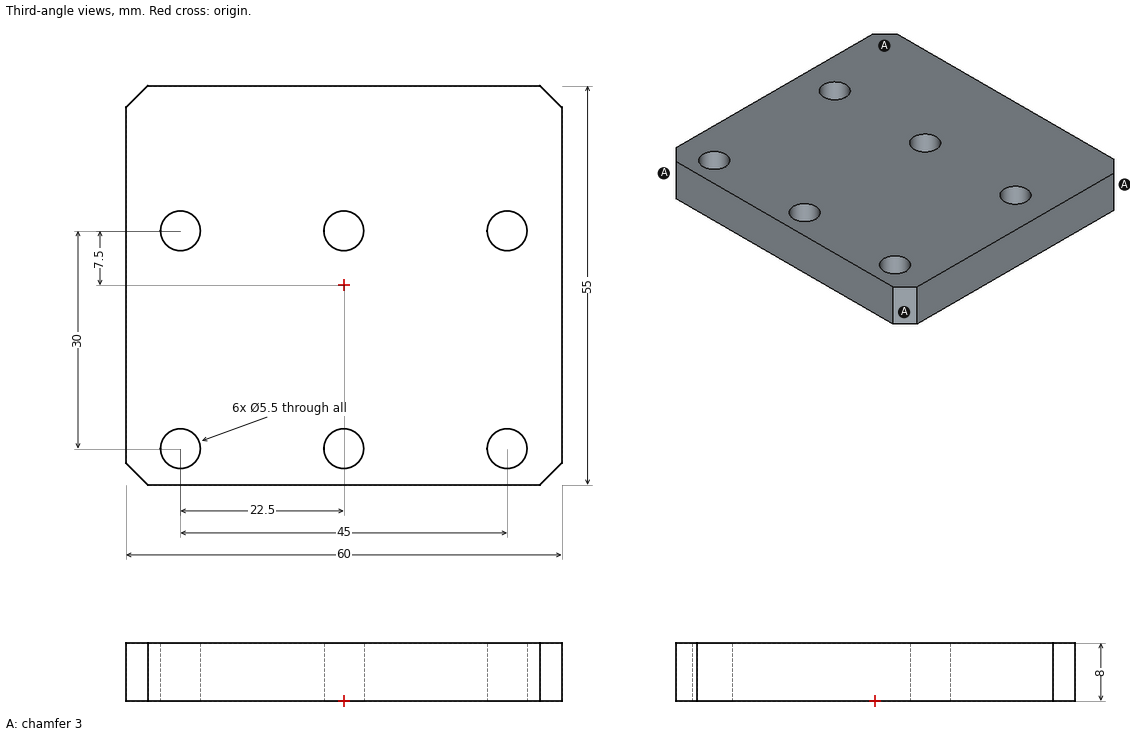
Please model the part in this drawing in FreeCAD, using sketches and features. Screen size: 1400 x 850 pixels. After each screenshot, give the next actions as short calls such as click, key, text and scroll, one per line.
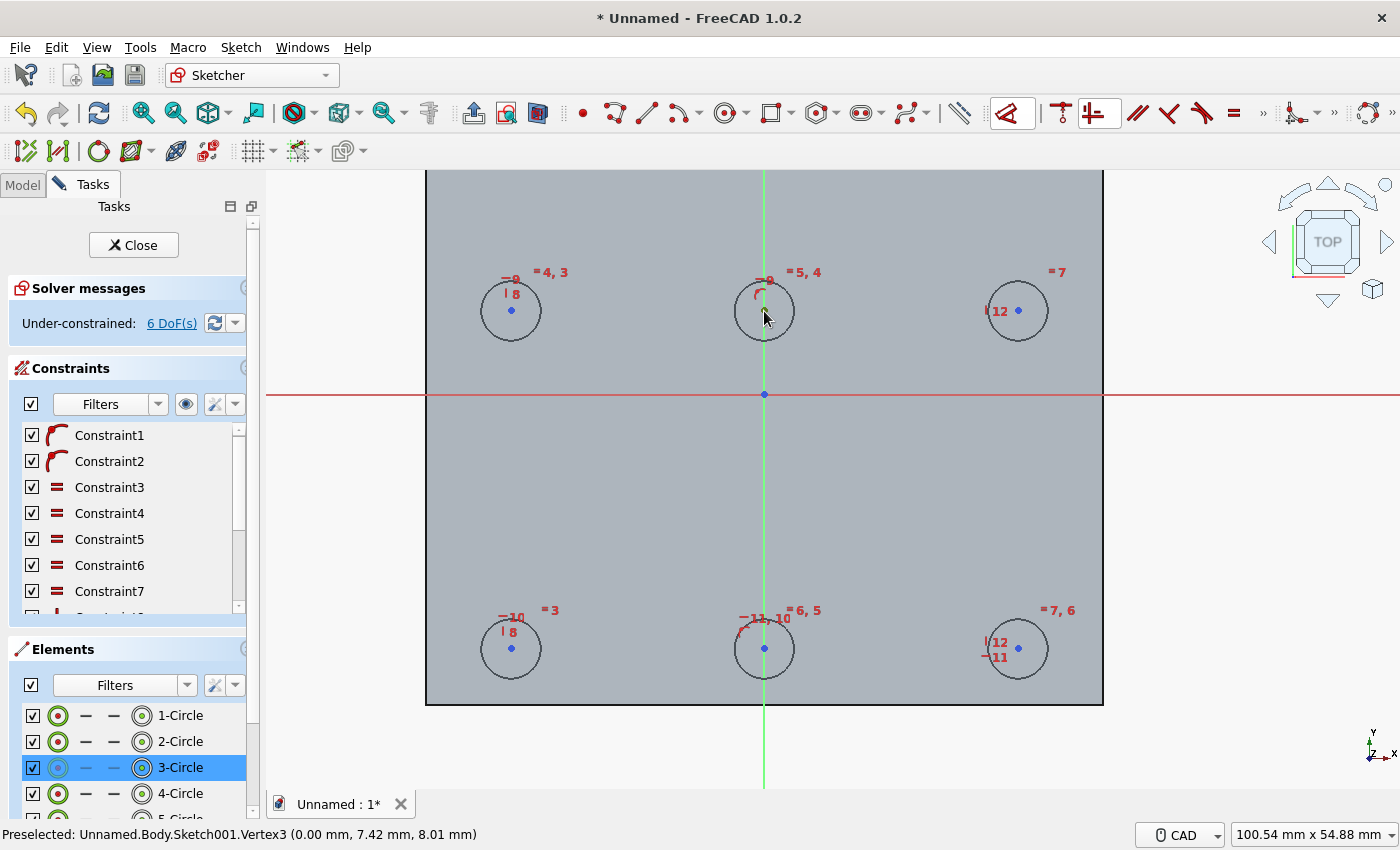
click(1018, 311)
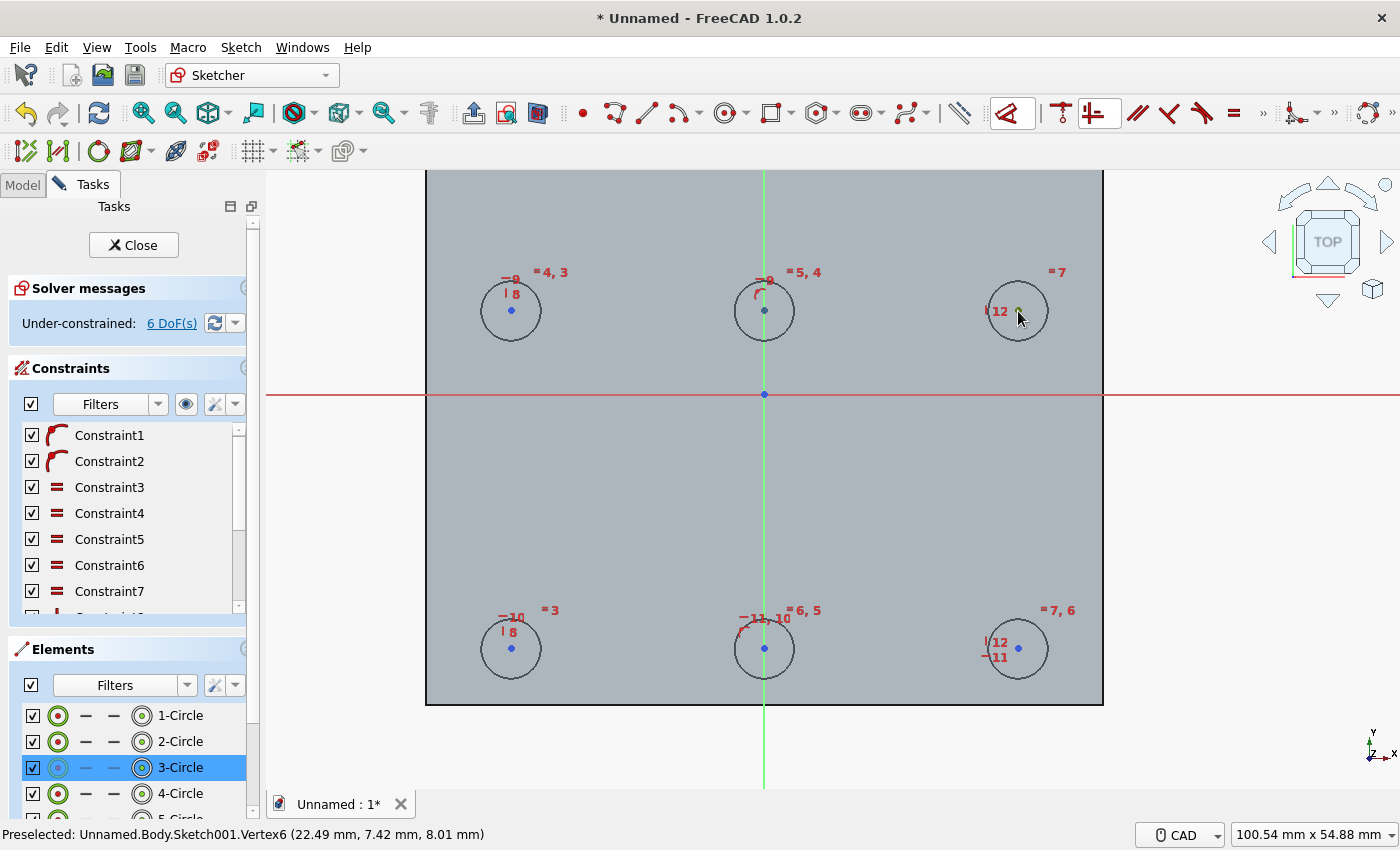
click(1116, 114)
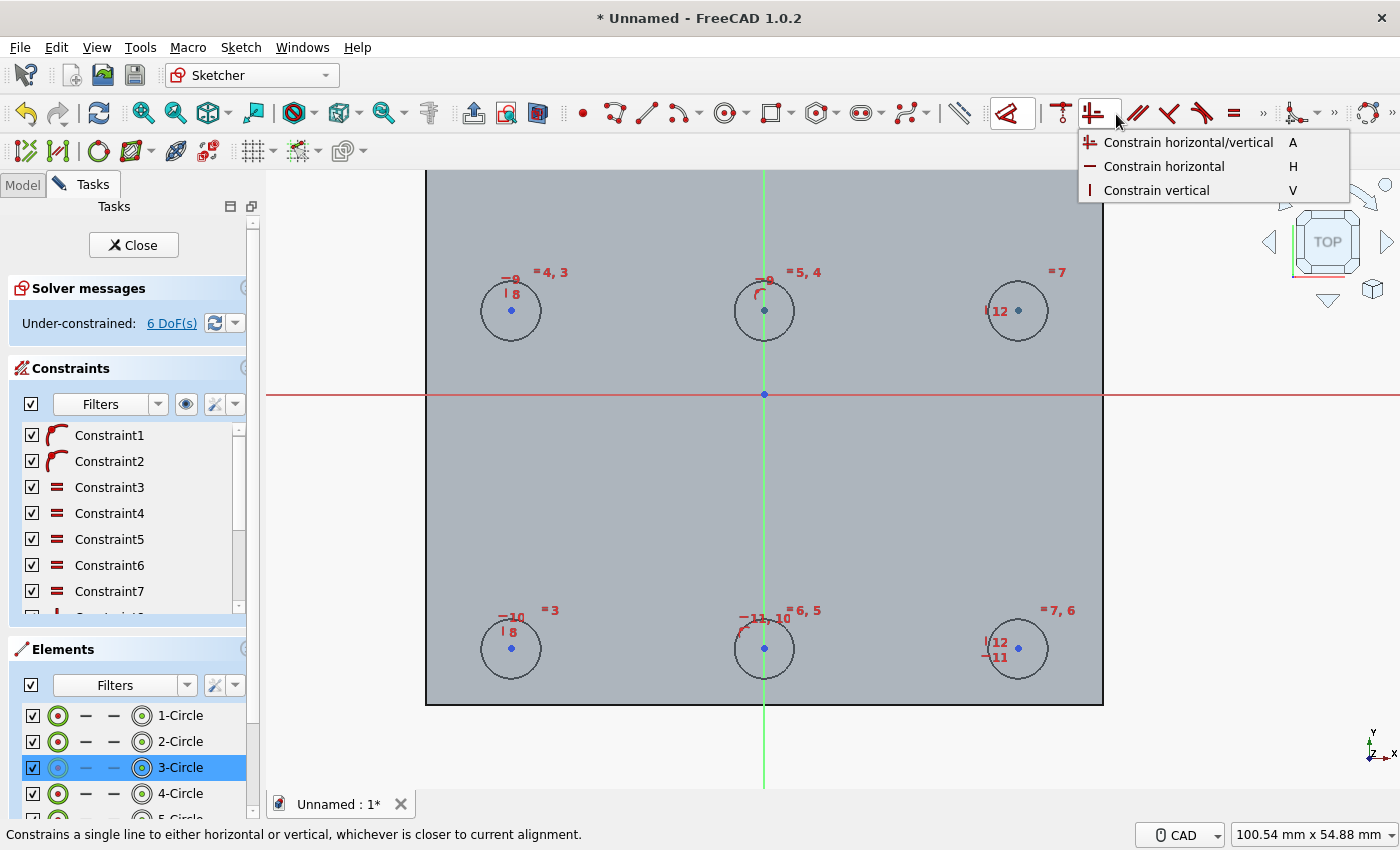
click(1214, 166)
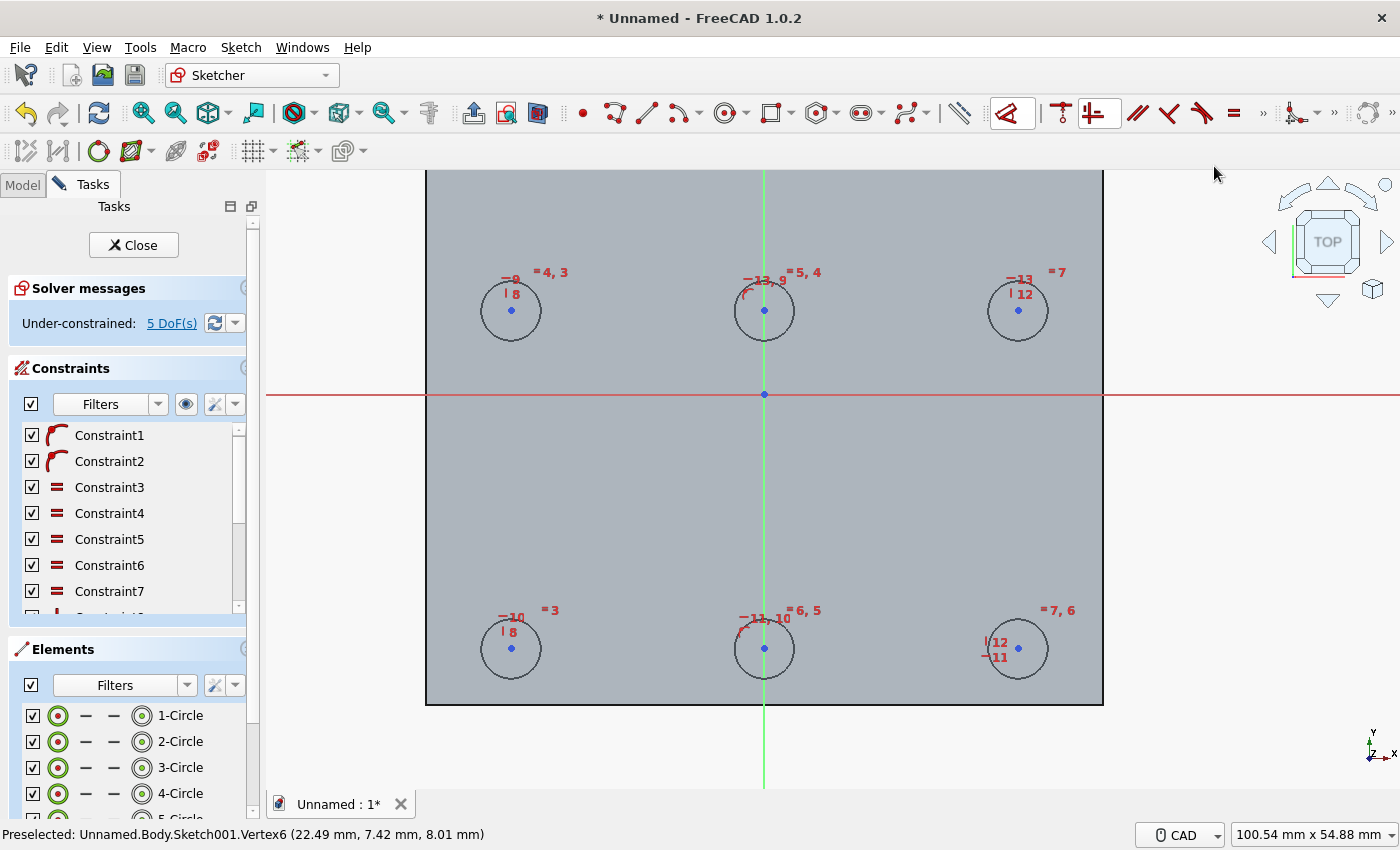
click(1006, 114)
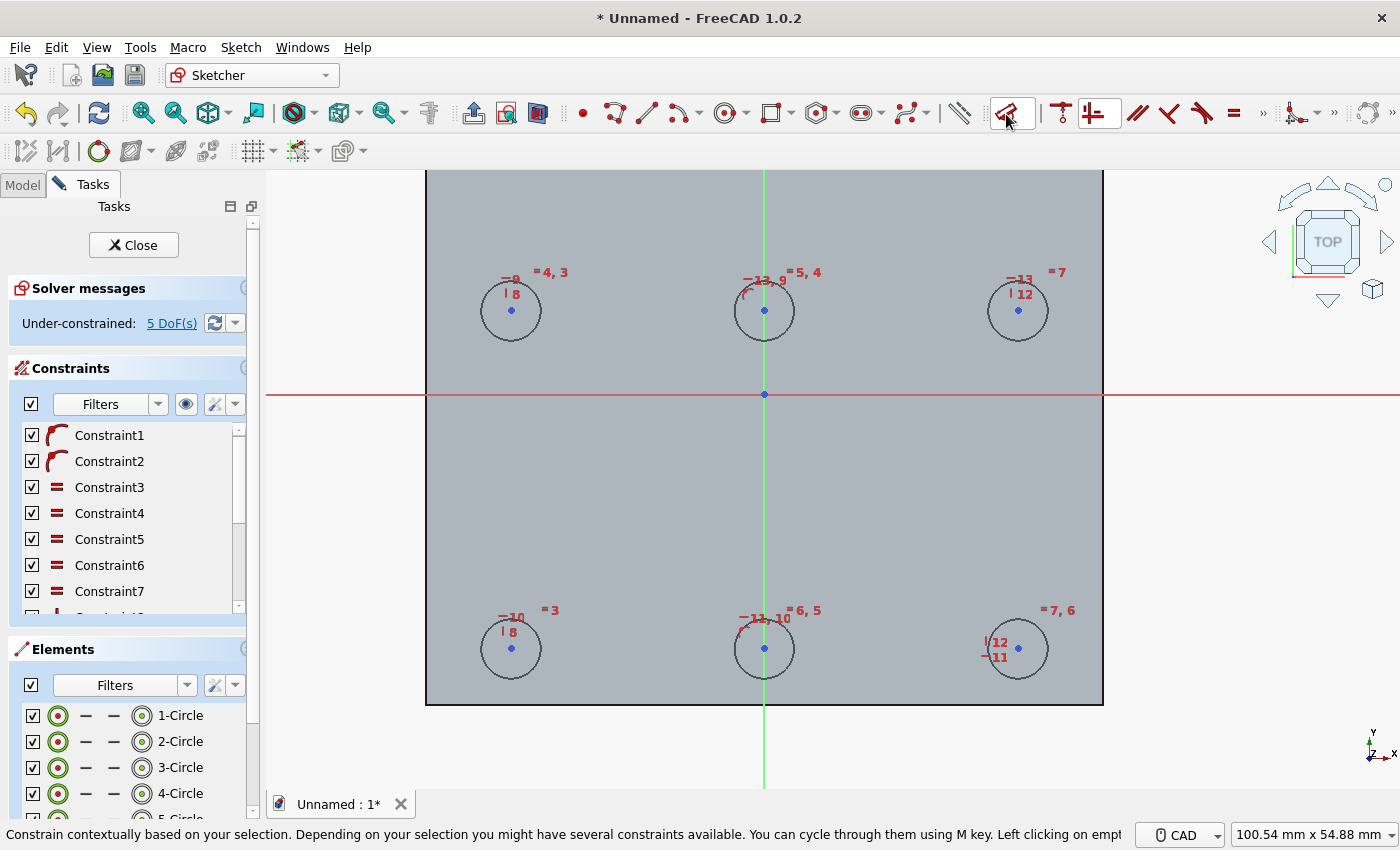
click(532, 628)
click(555, 605)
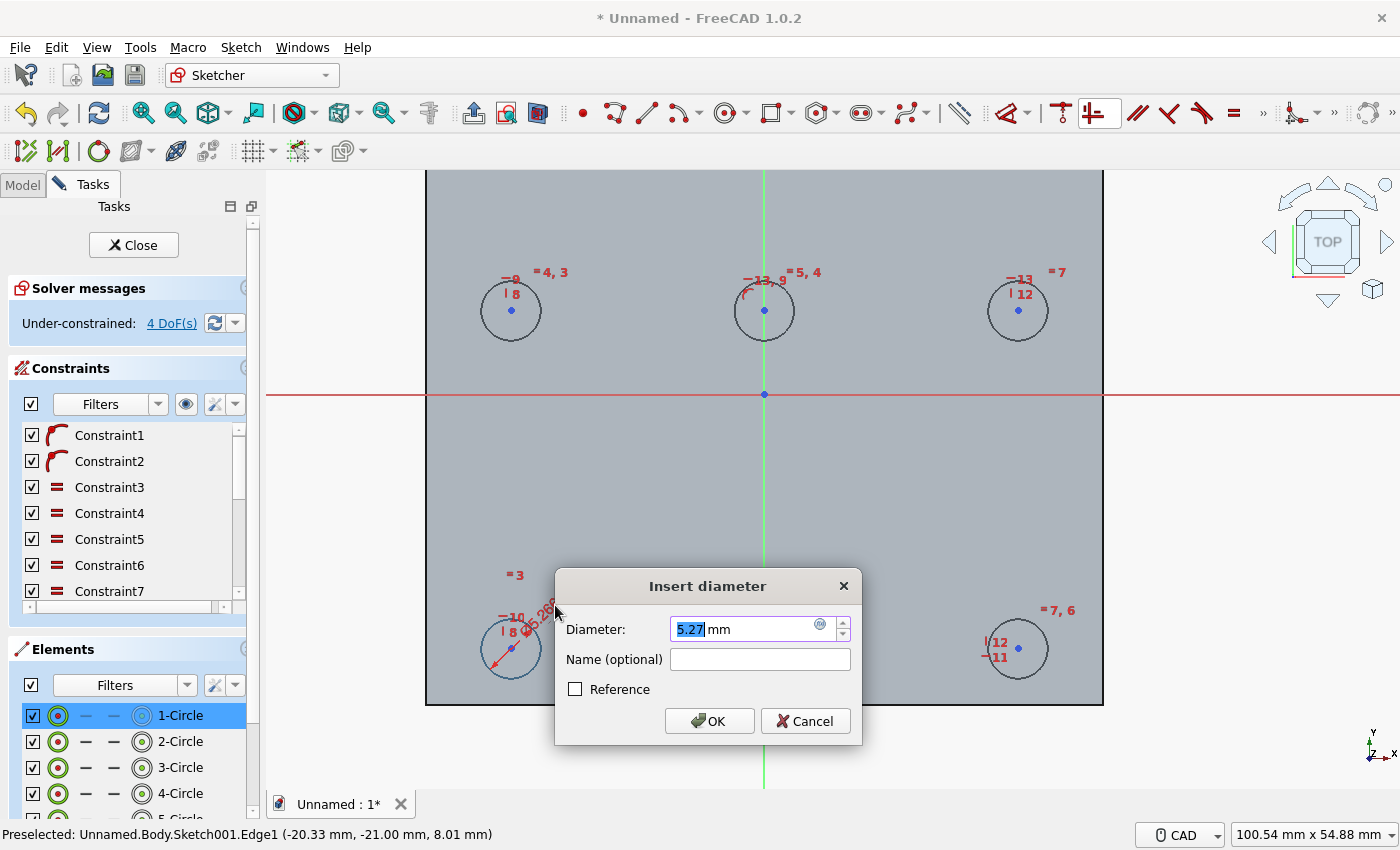
text(5.5)
key(Return)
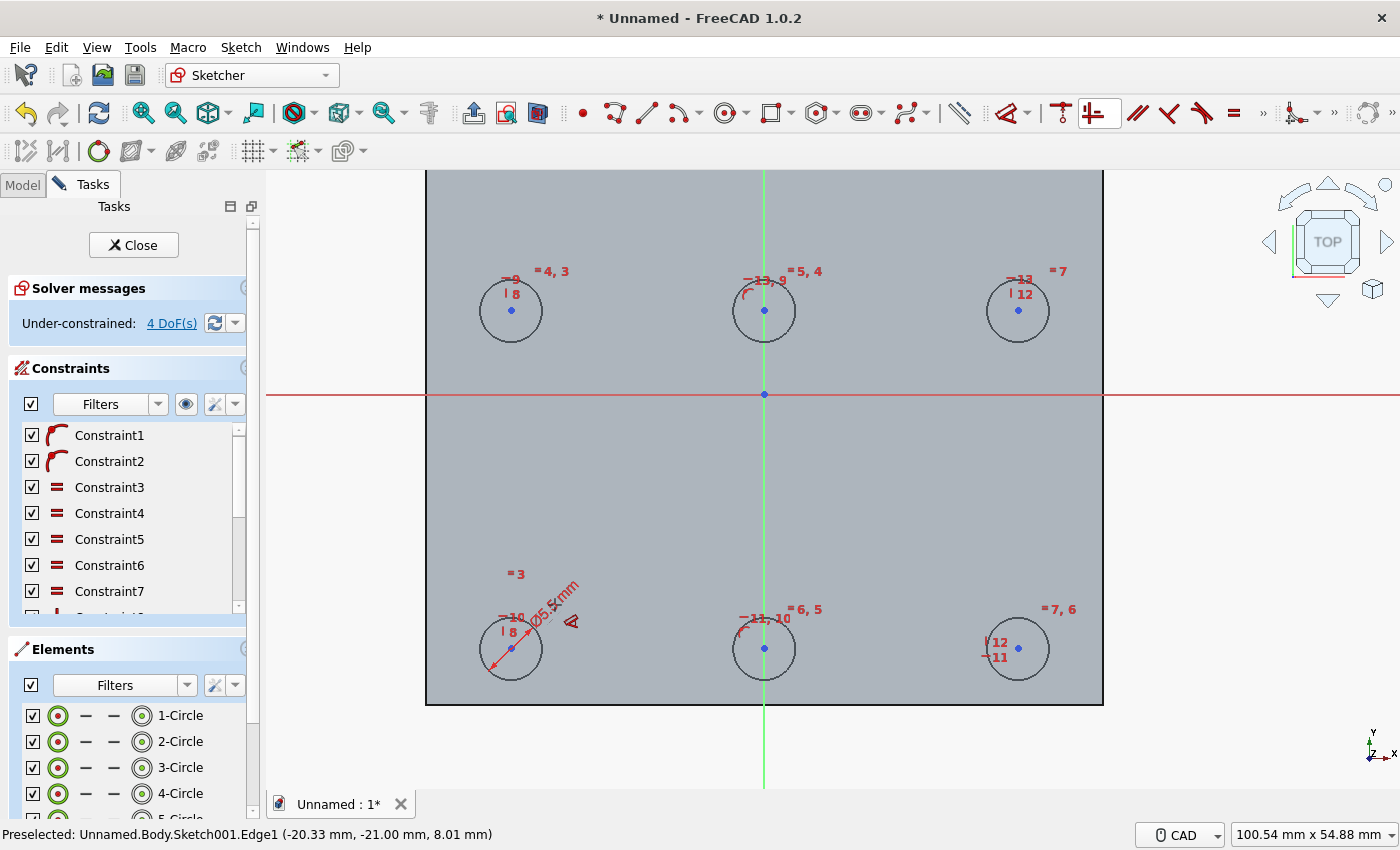
click(511, 311)
click(477, 353)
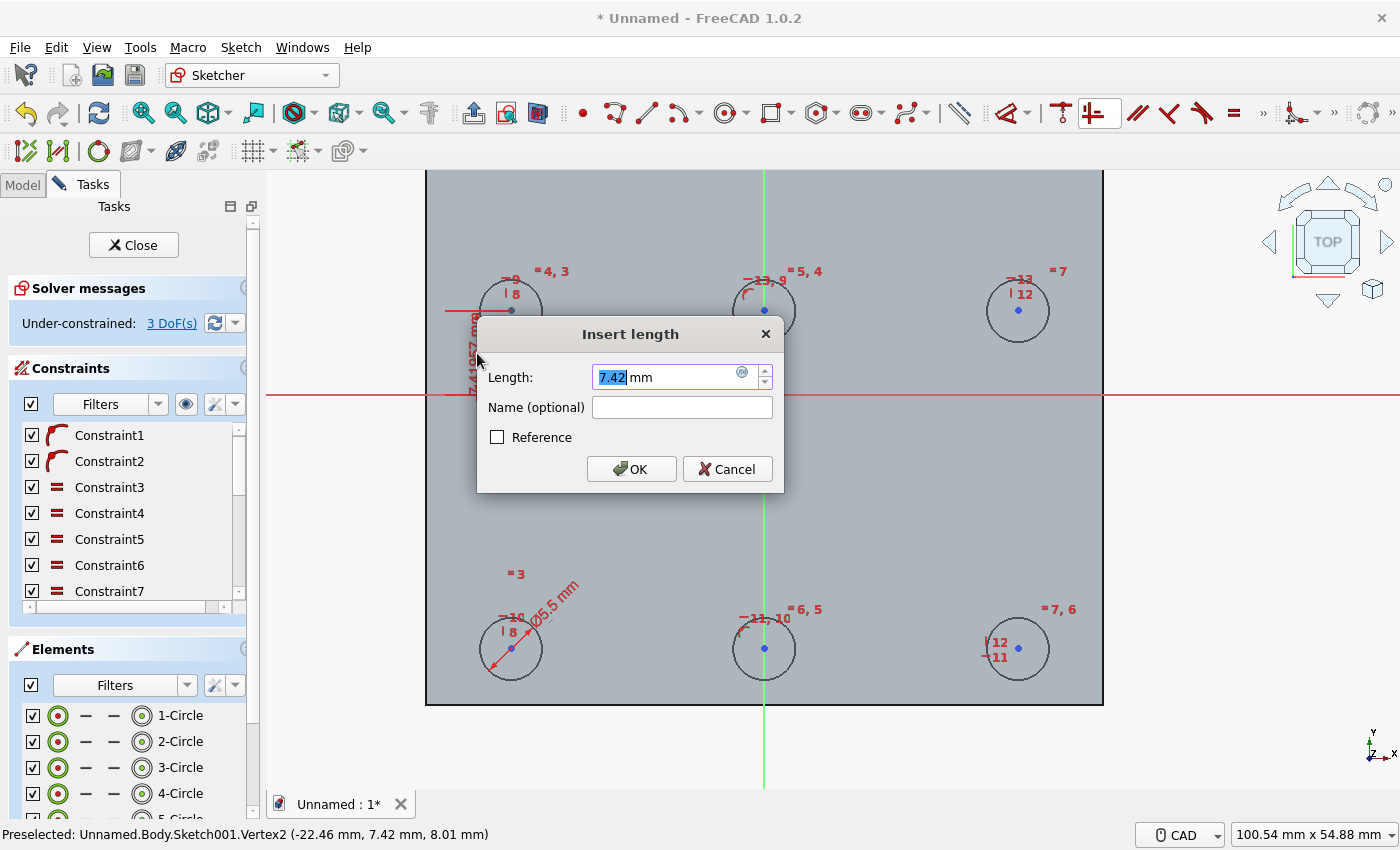
text(7.5)
key(Return)